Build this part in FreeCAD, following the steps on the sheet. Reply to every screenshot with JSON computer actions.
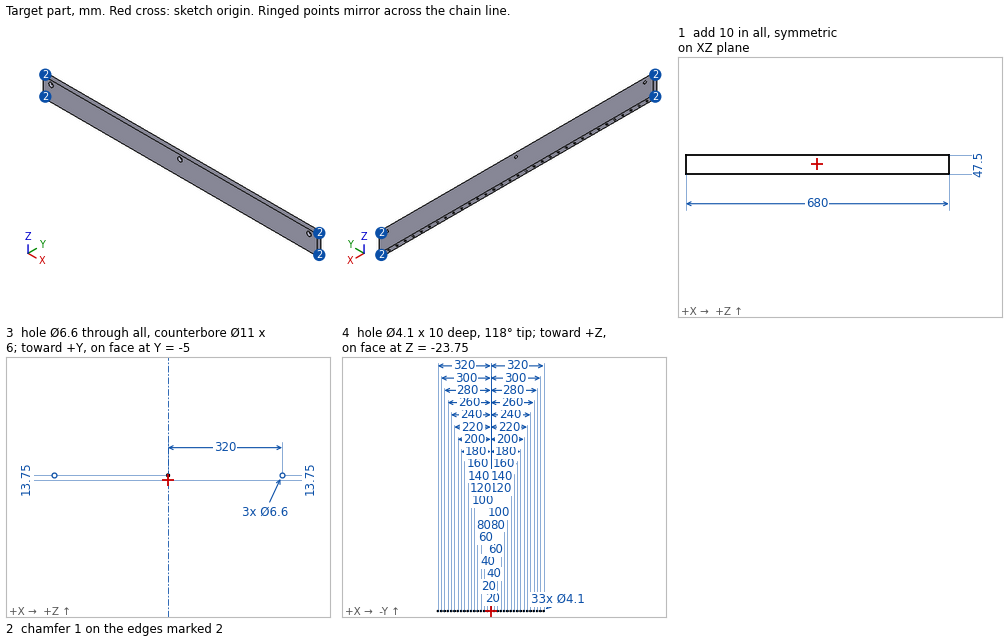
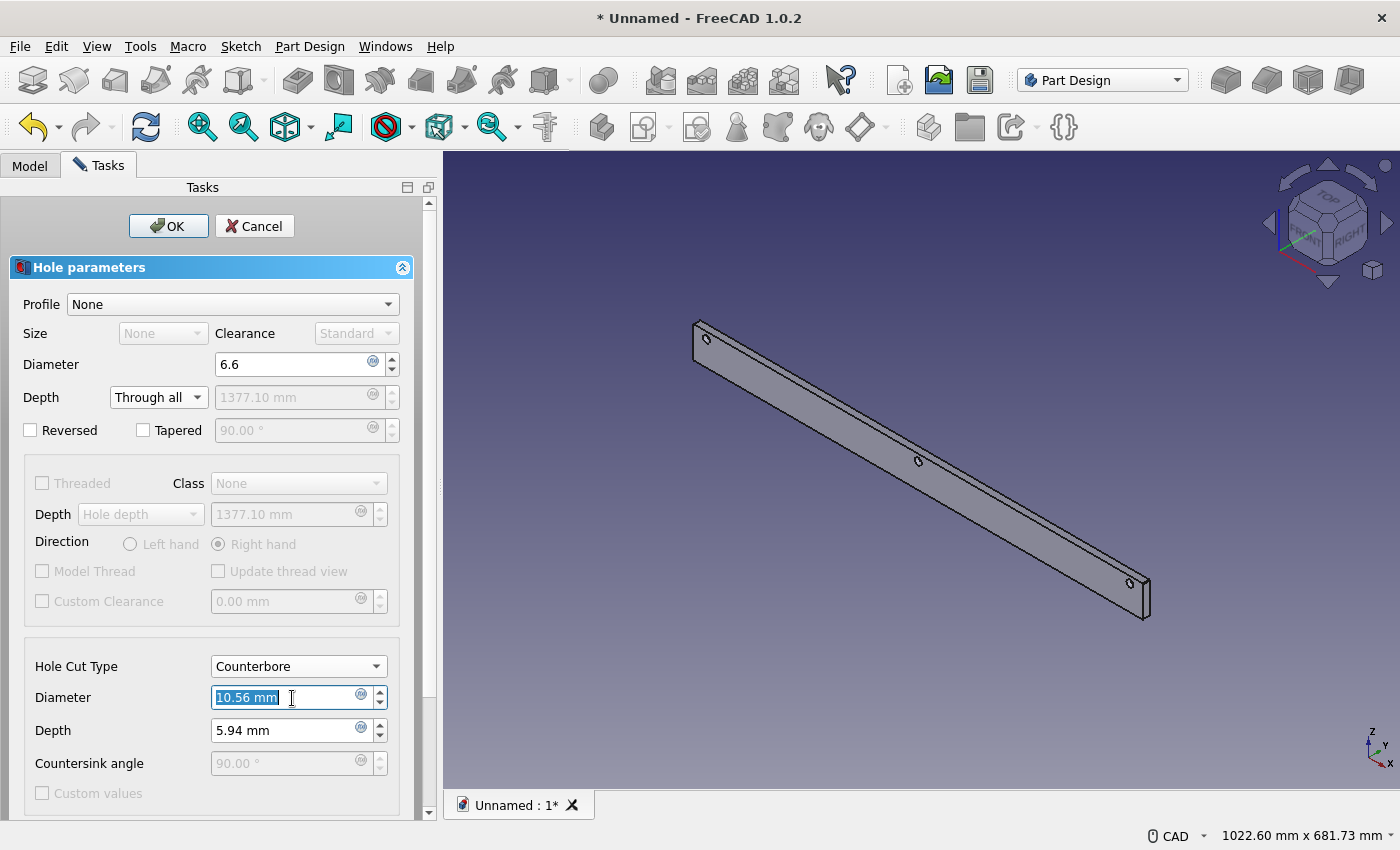
{"action": "type", "text": "11"}
{"action": "key", "text": "Tab"}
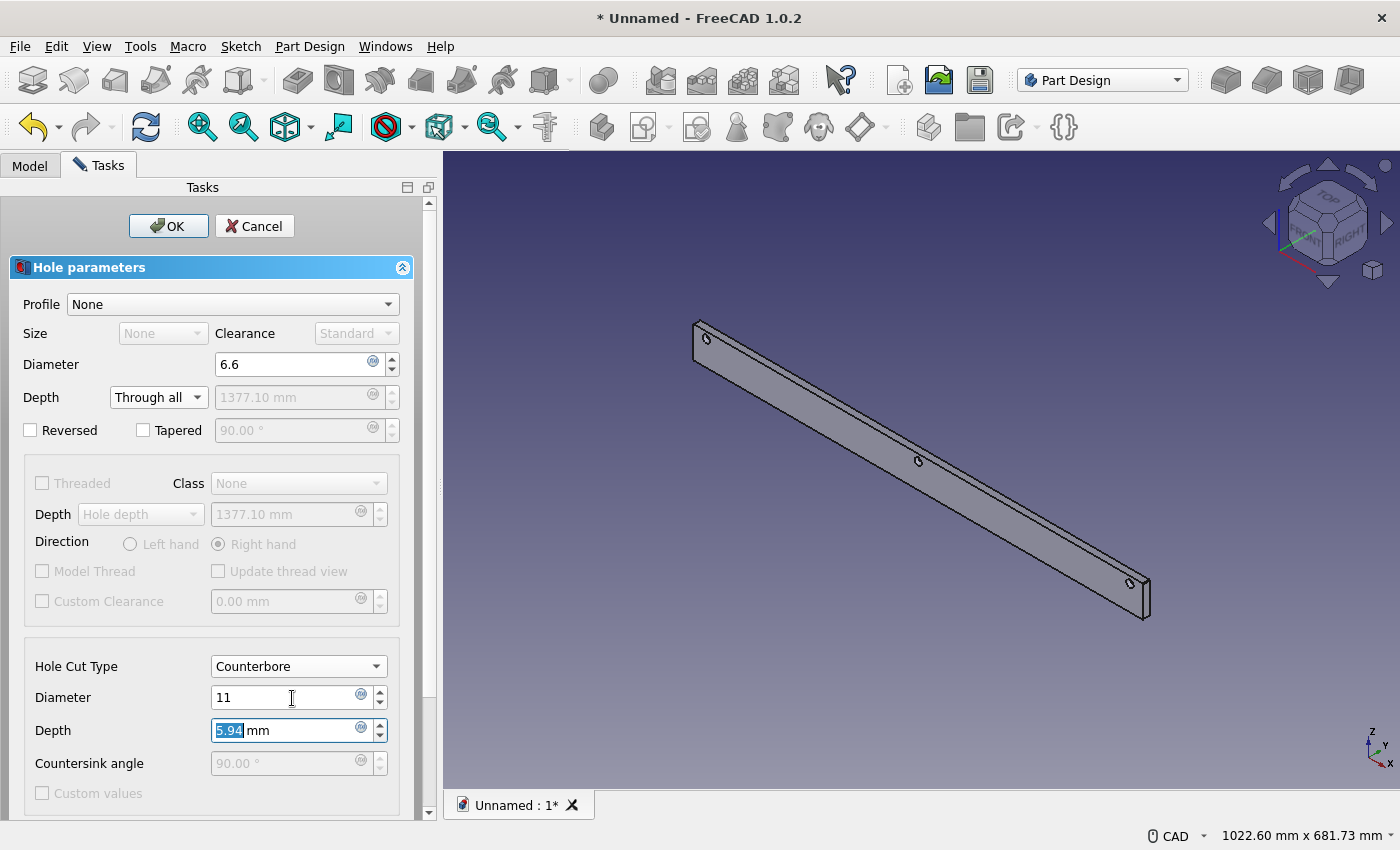
{"action": "type", "text": "6"}
{"action": "key", "text": "Tab"}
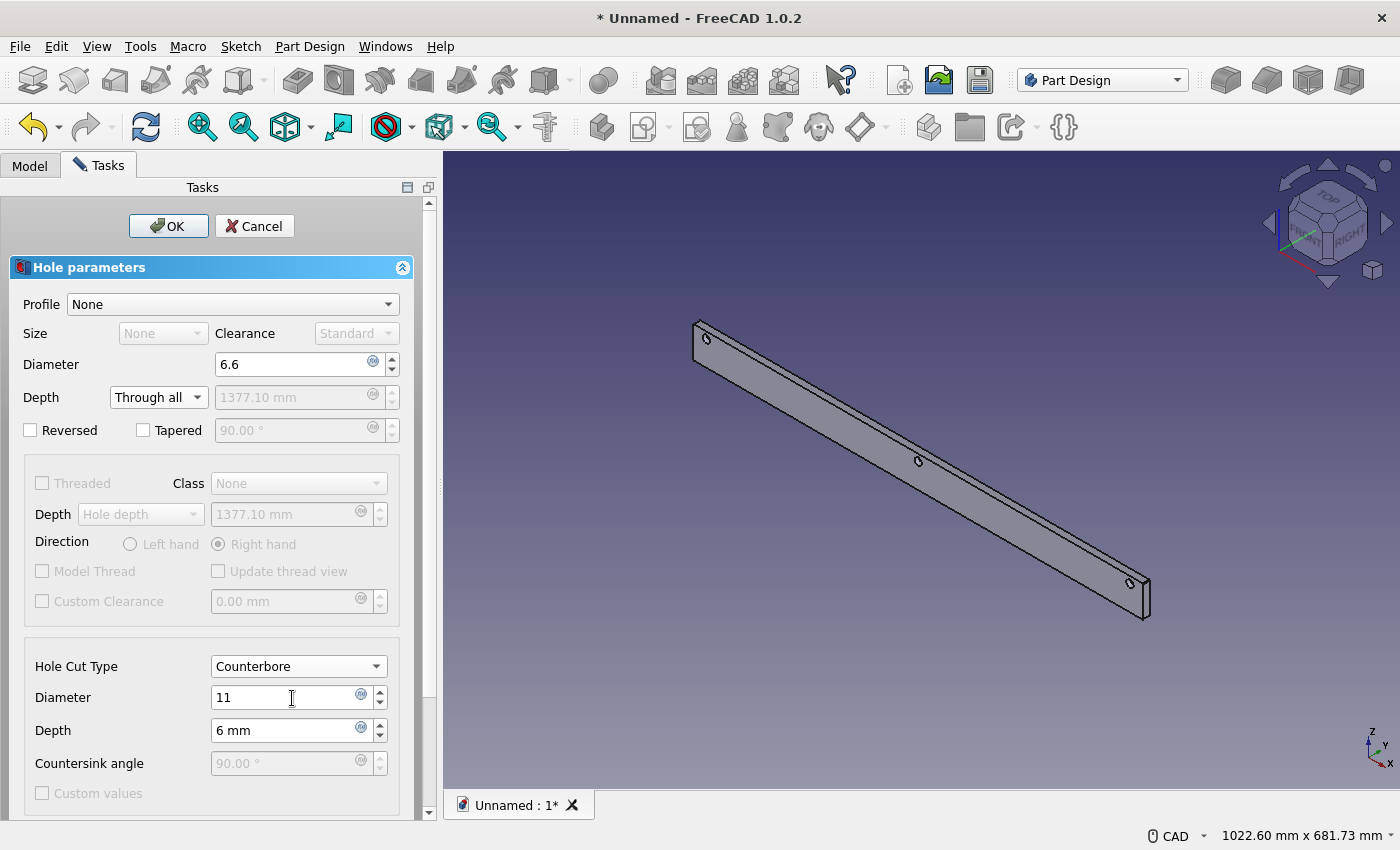
{"action": "left_click", "coordinate": [169, 226]}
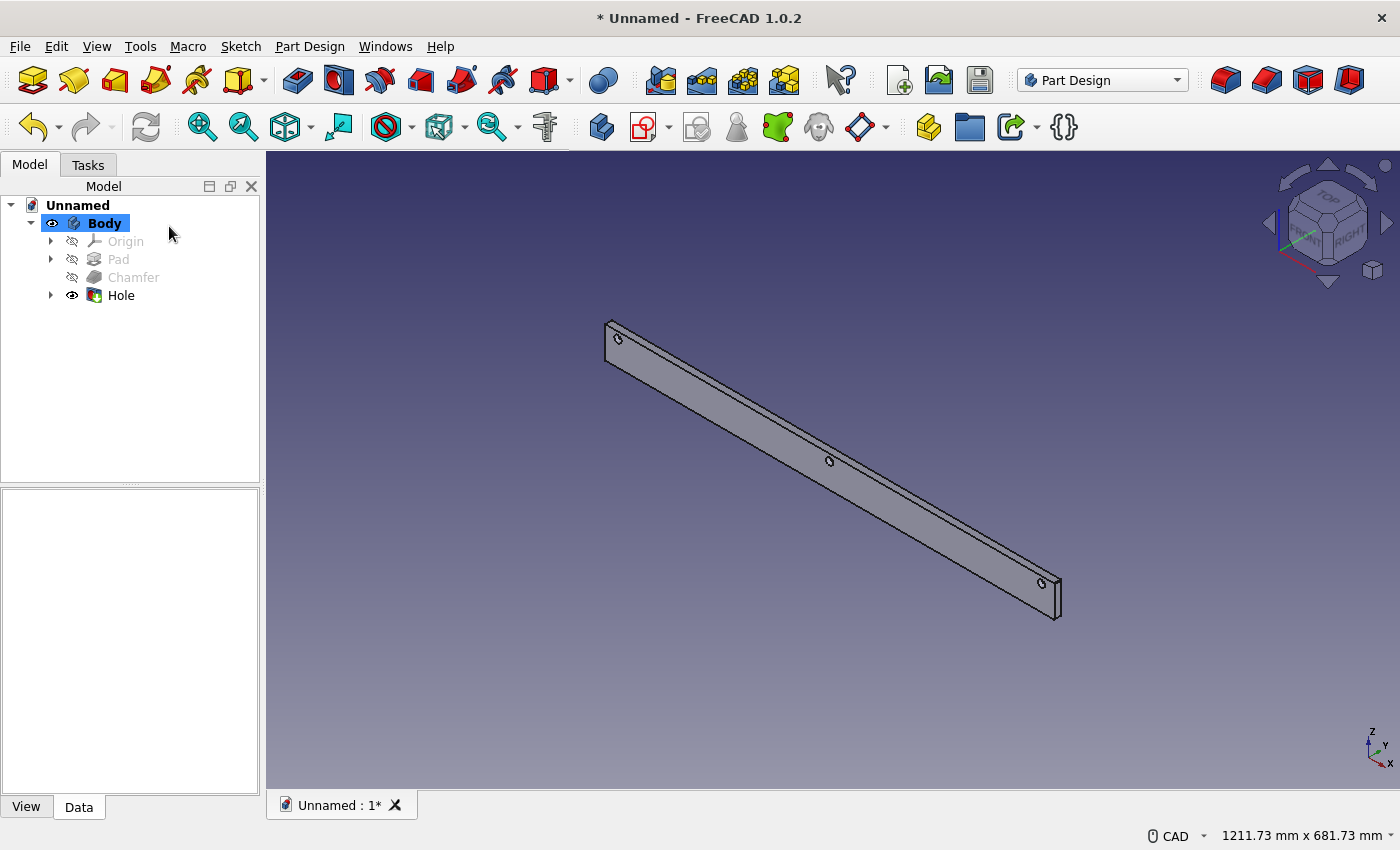
{"action": "key", "text": "5"}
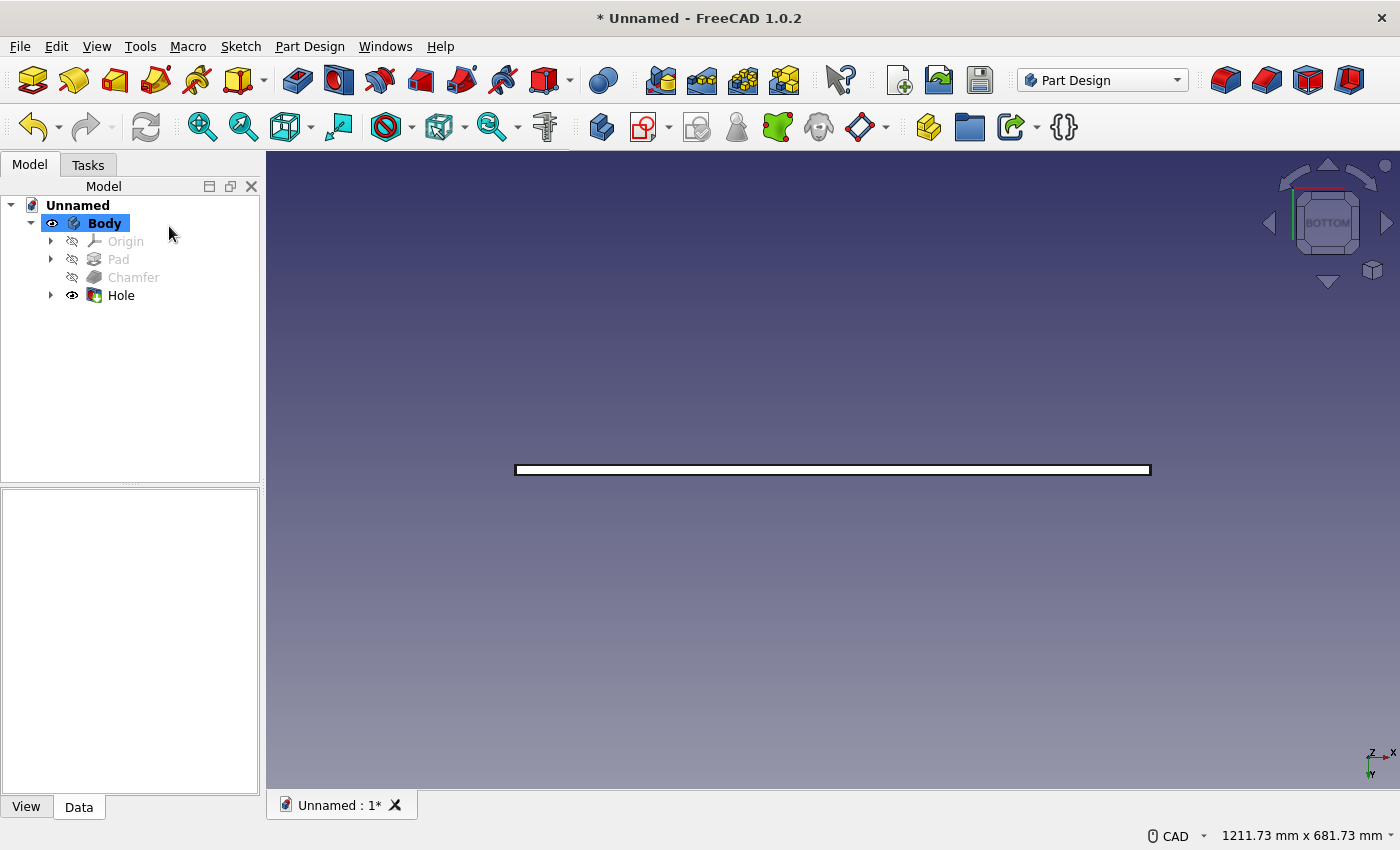
{"action": "scroll", "coordinate": [1105, 469], "scroll_direction": "up", "scroll_amount": 5}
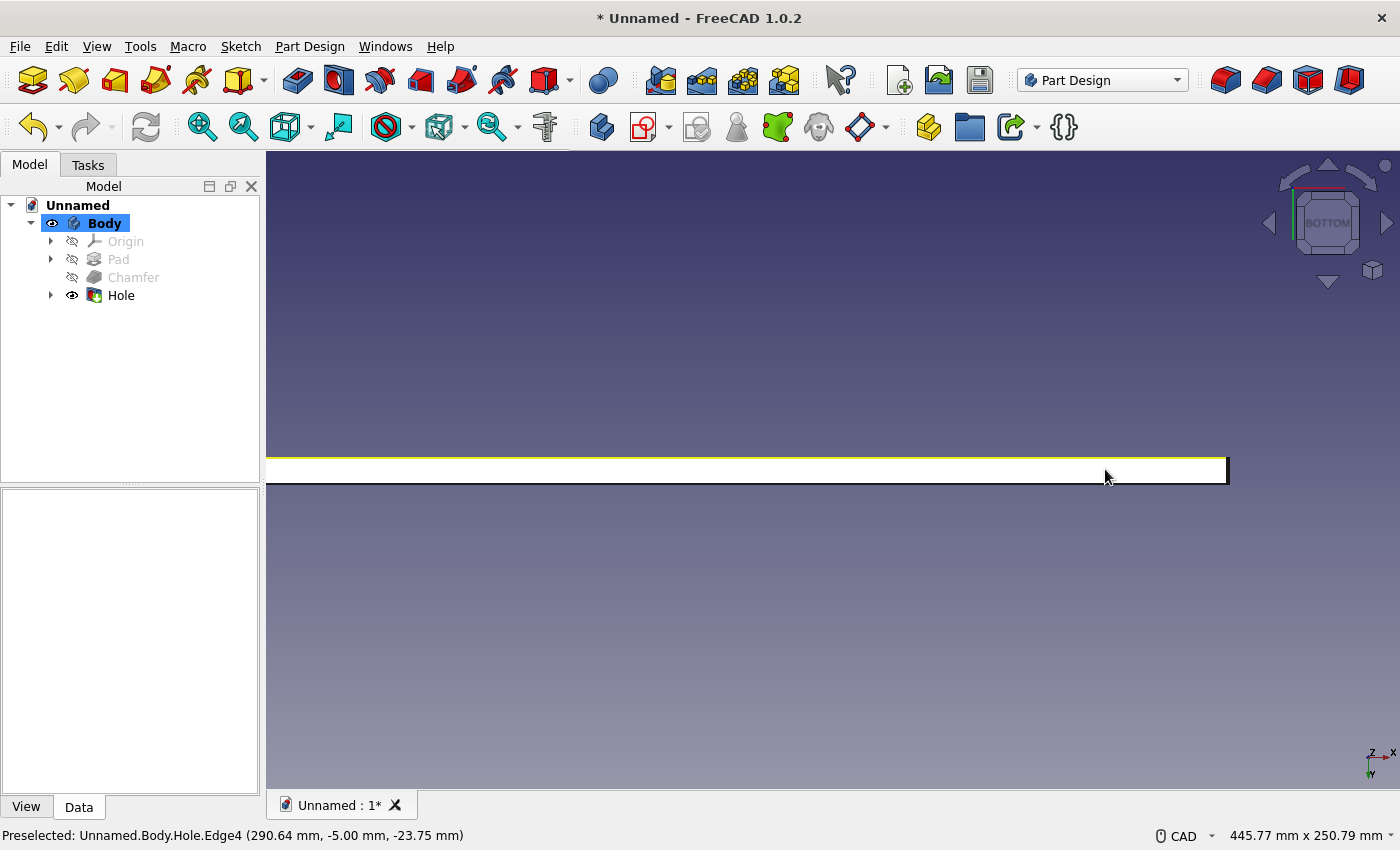
{"action": "left_click", "coordinate": [1104, 470]}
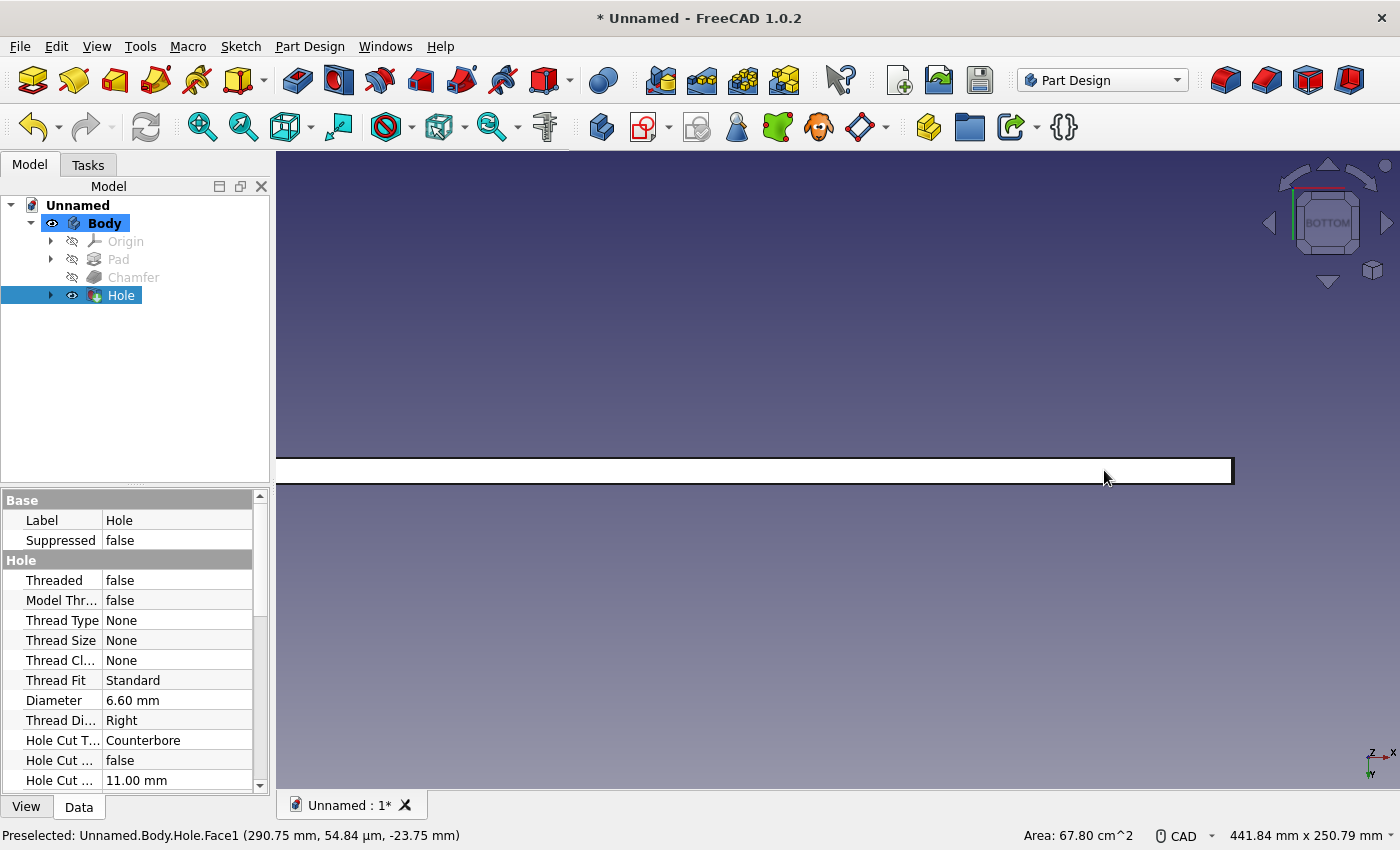
{"action": "left_click", "coordinate": [642, 128]}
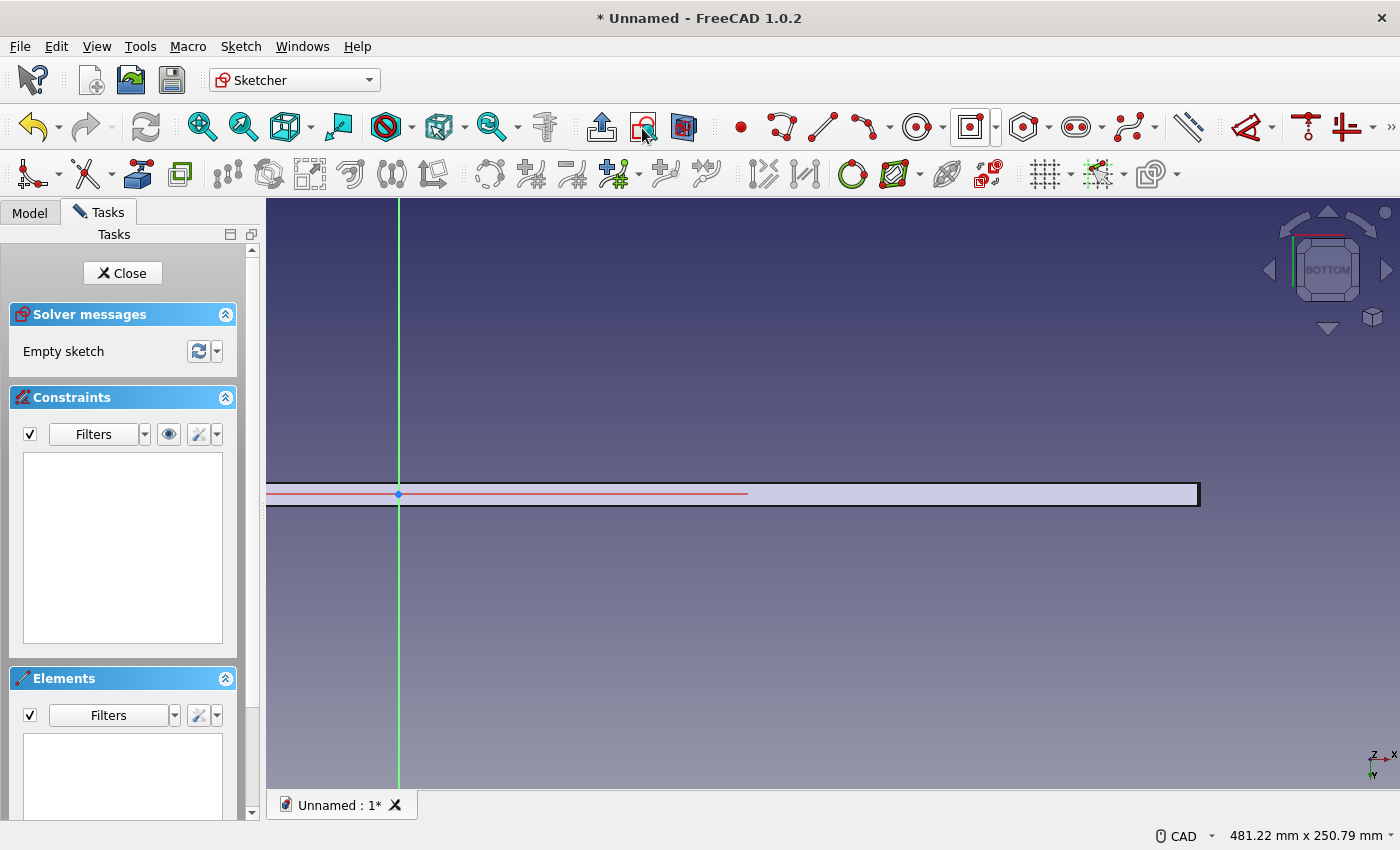
{"action": "scroll", "coordinate": [1063, 493], "scroll_direction": "down", "scroll_amount": 4}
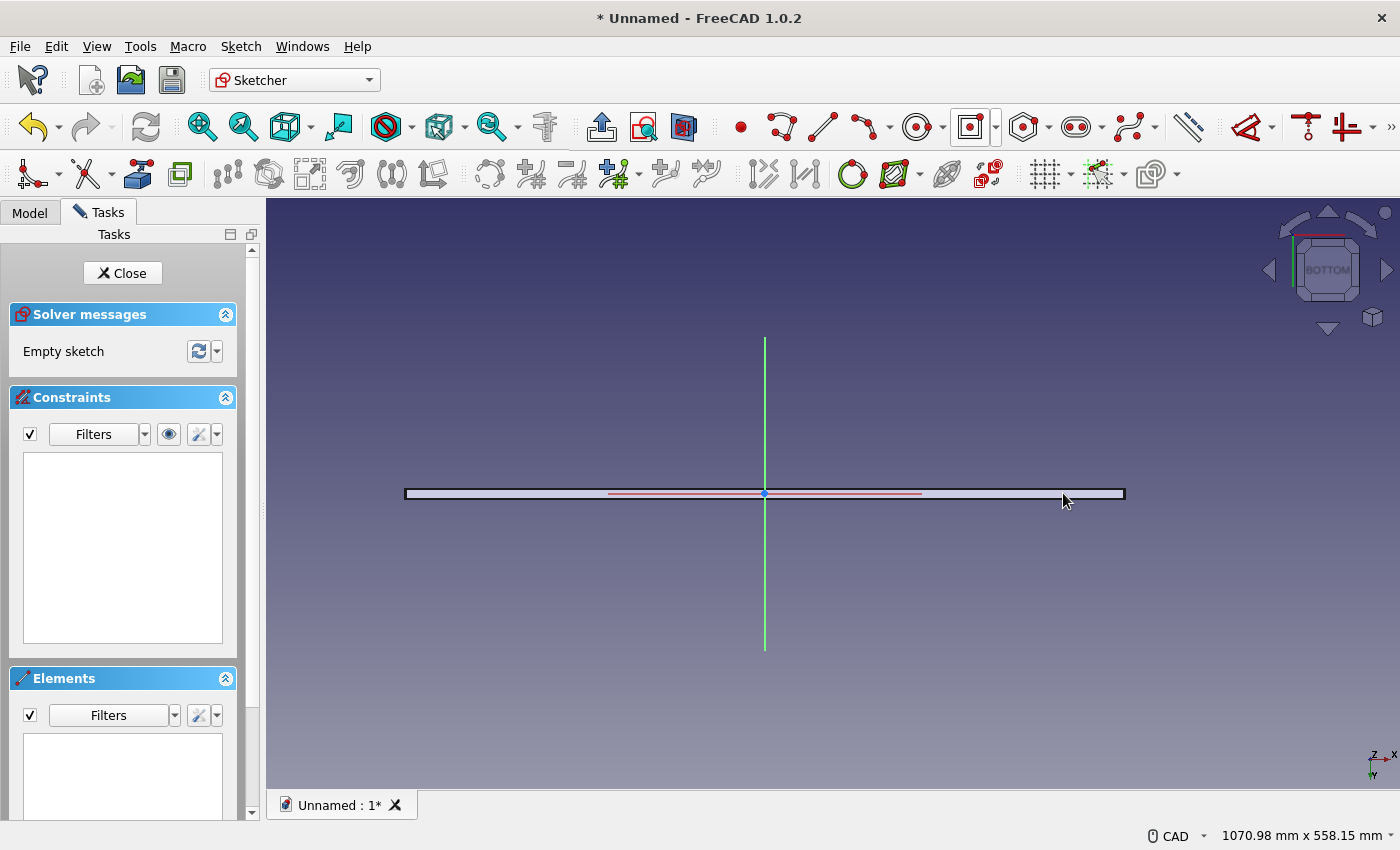
{"action": "left_click", "coordinate": [916, 128]}